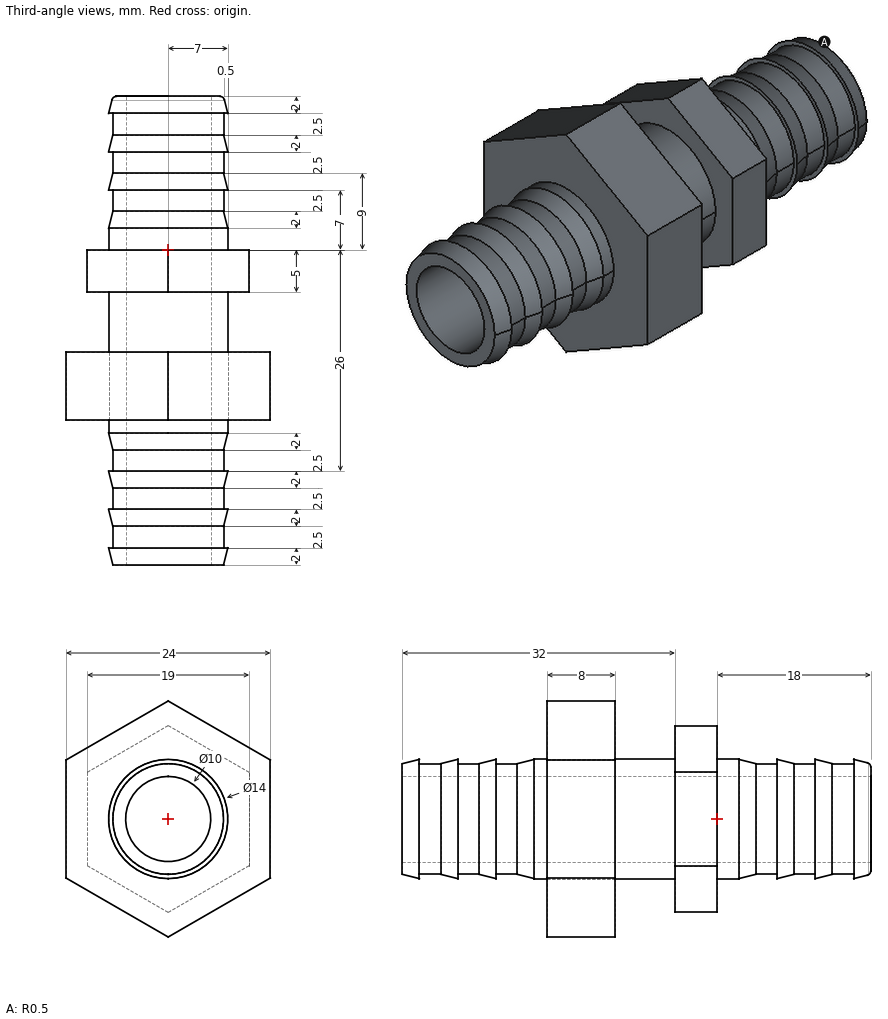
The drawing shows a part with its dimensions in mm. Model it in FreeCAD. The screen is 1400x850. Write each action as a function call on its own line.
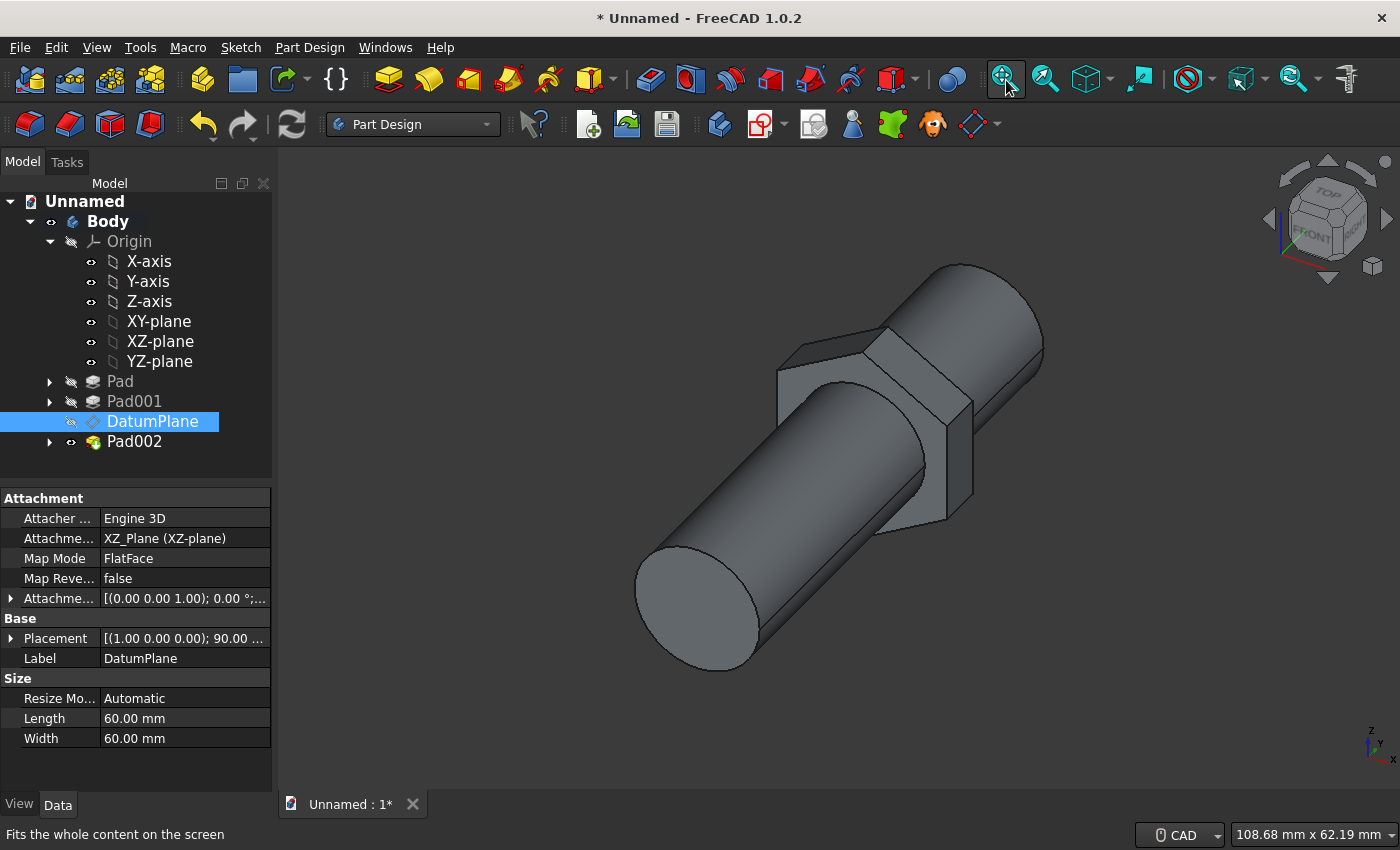
key(4)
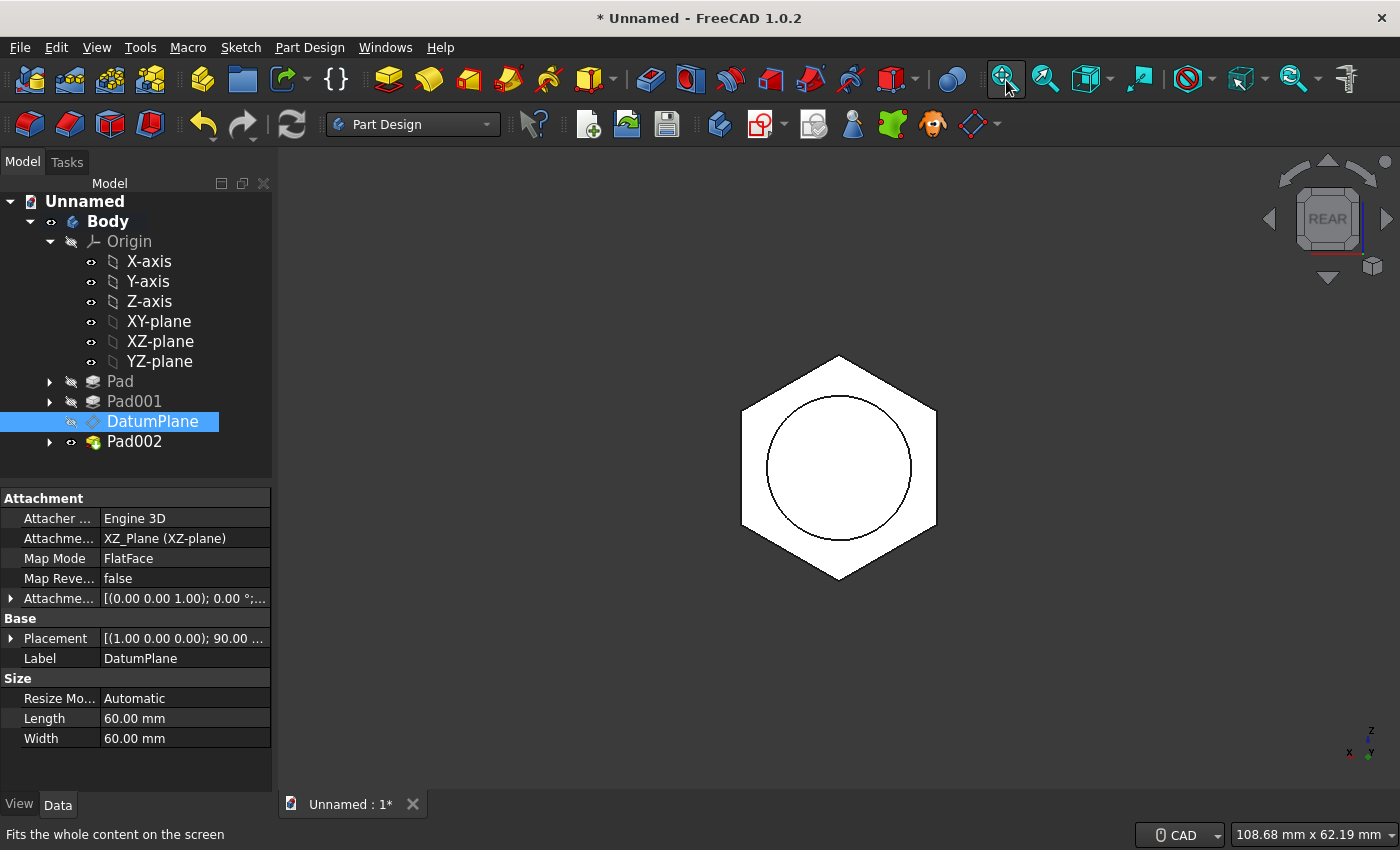
click(1006, 80)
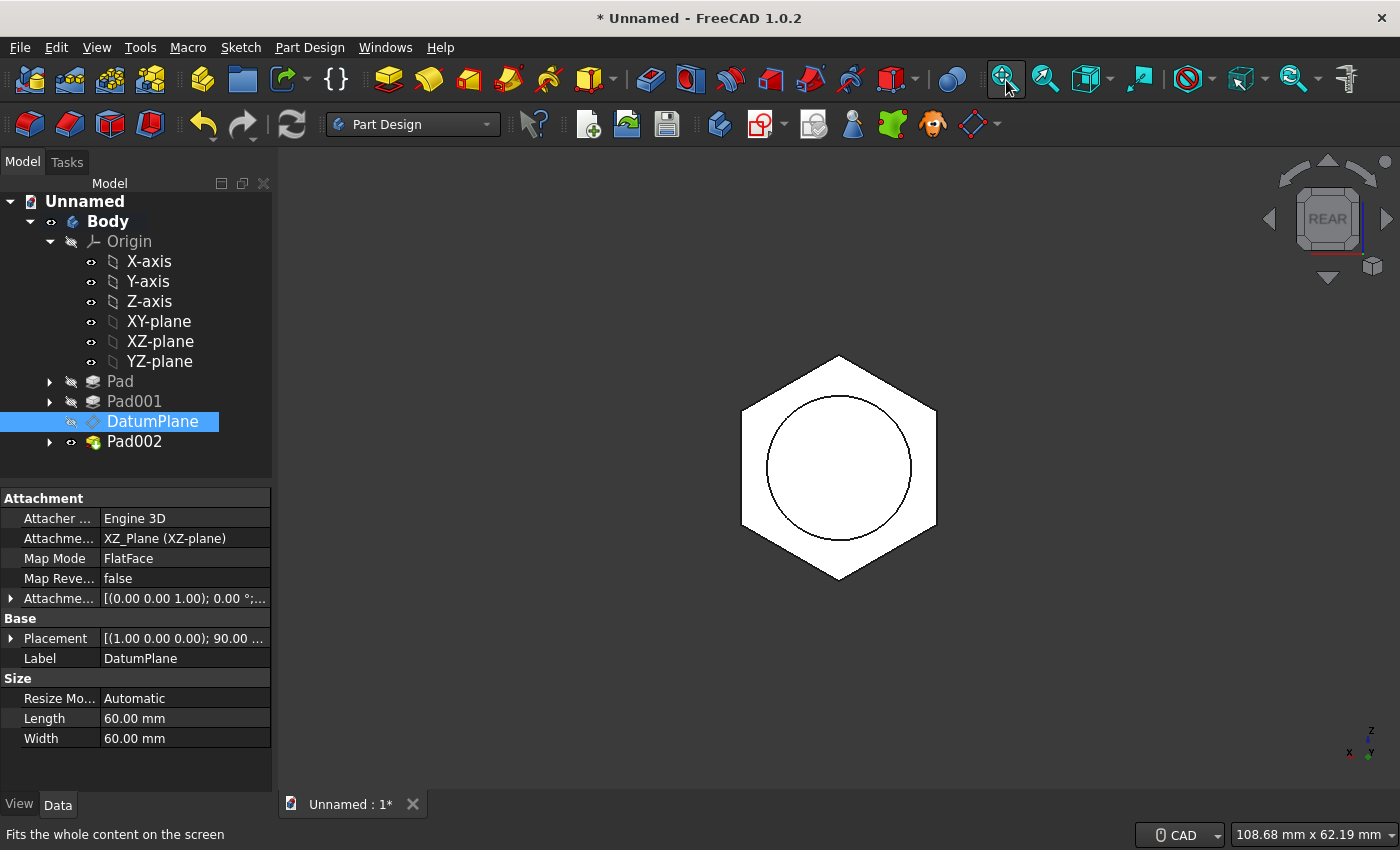
click(839, 467)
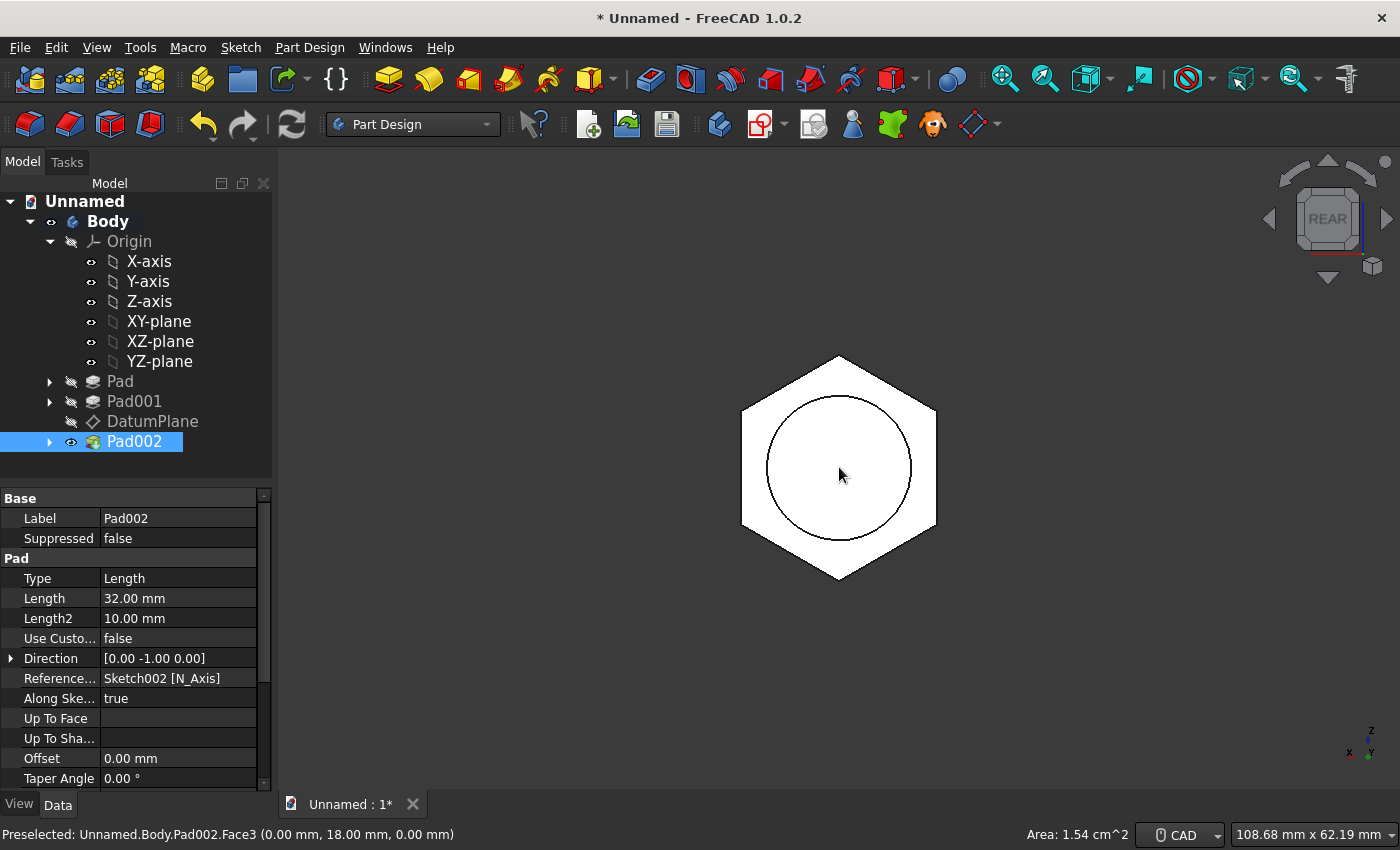
click(760, 124)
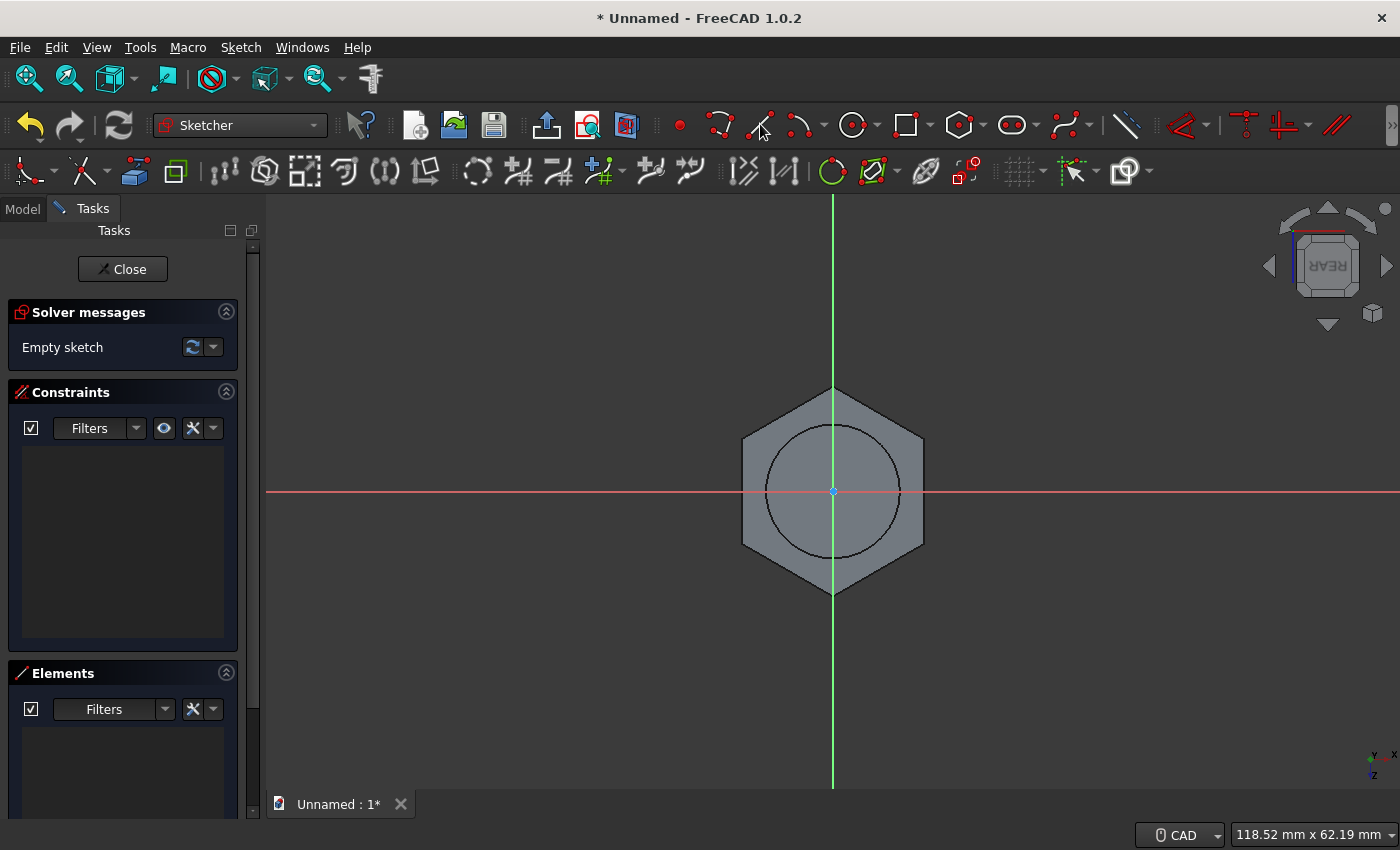
scroll(855, 492, up, 7)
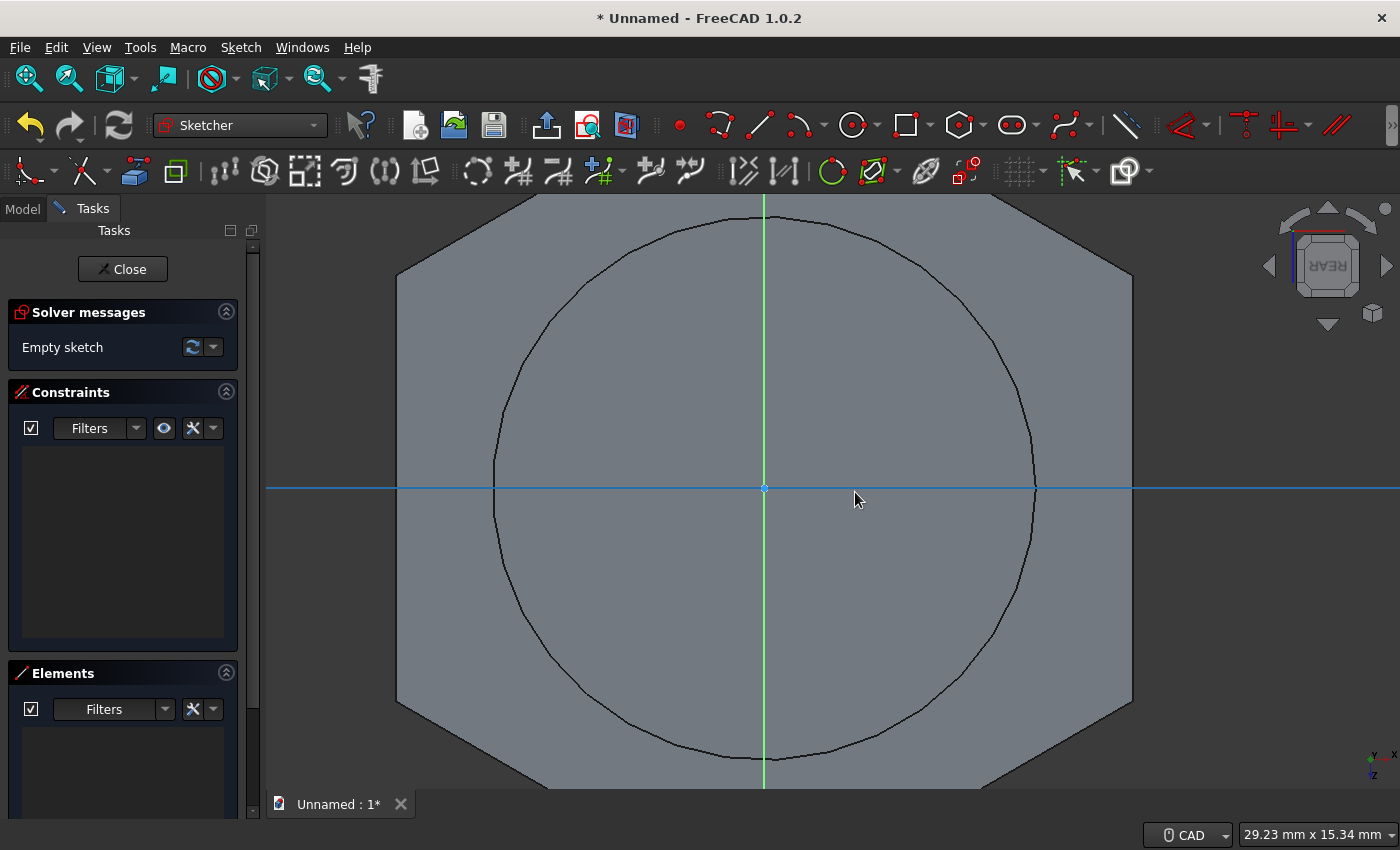
click(854, 126)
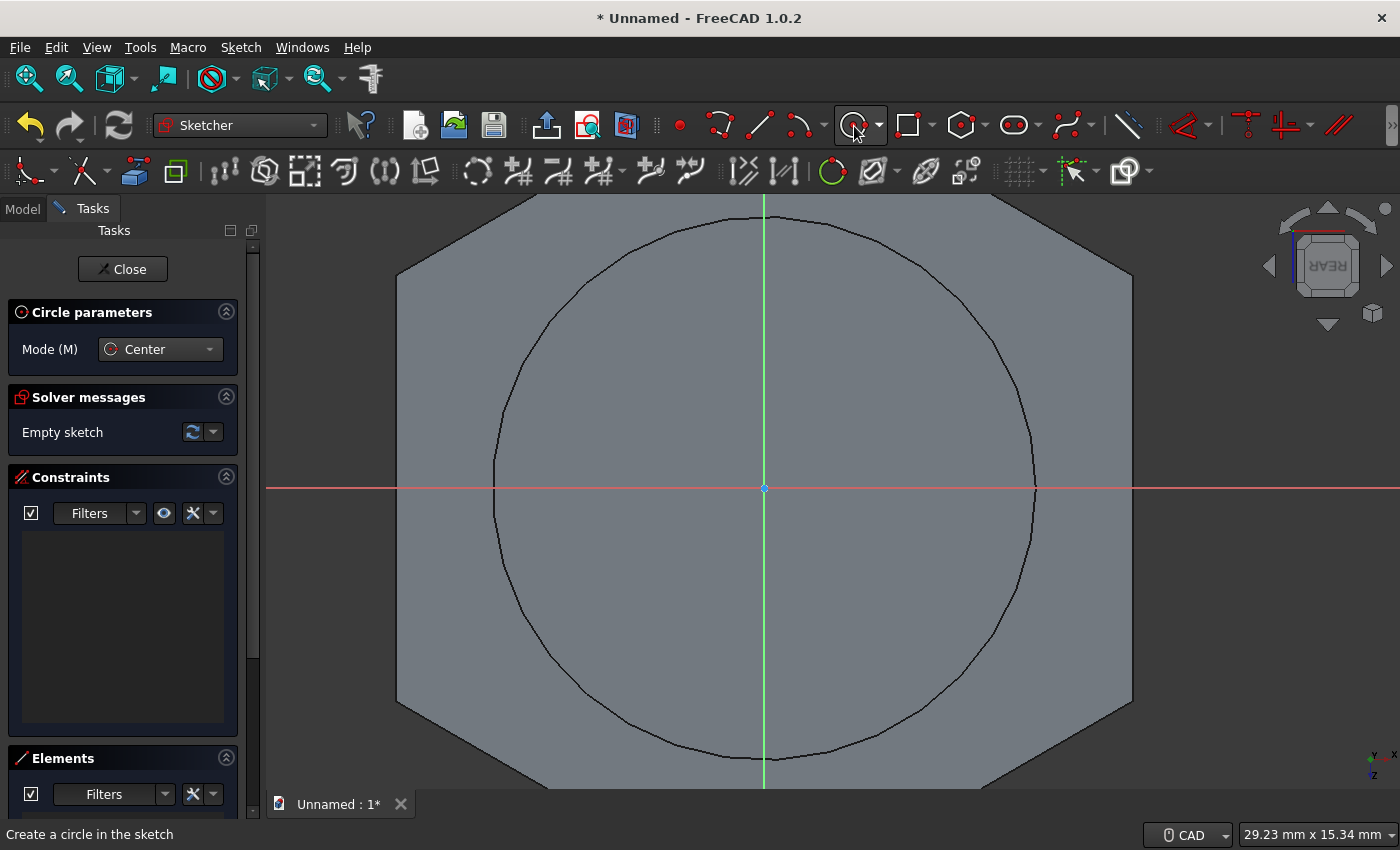
click(764, 488)
move(901, 351)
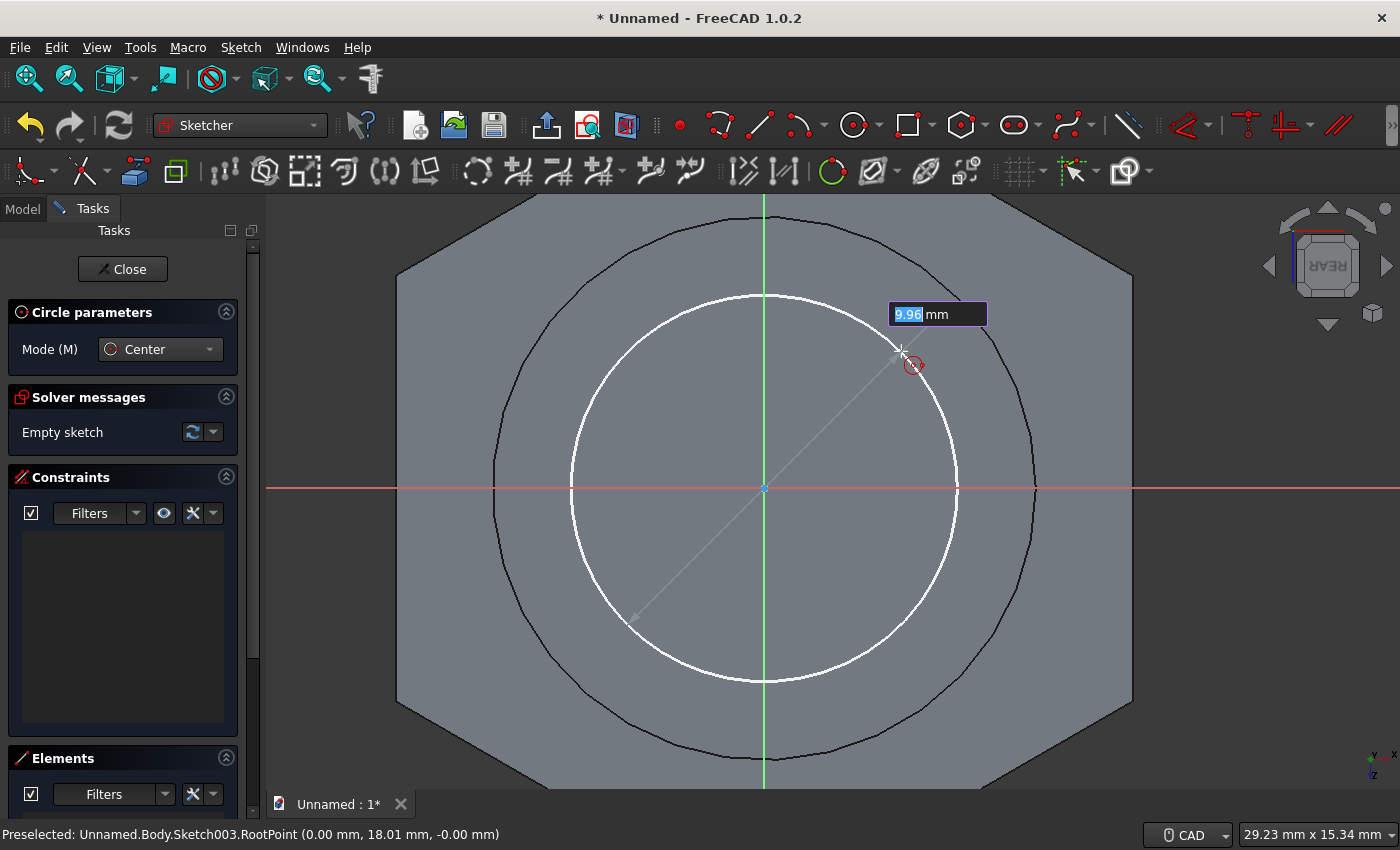
text(10)
key(Return)
key(Escape)